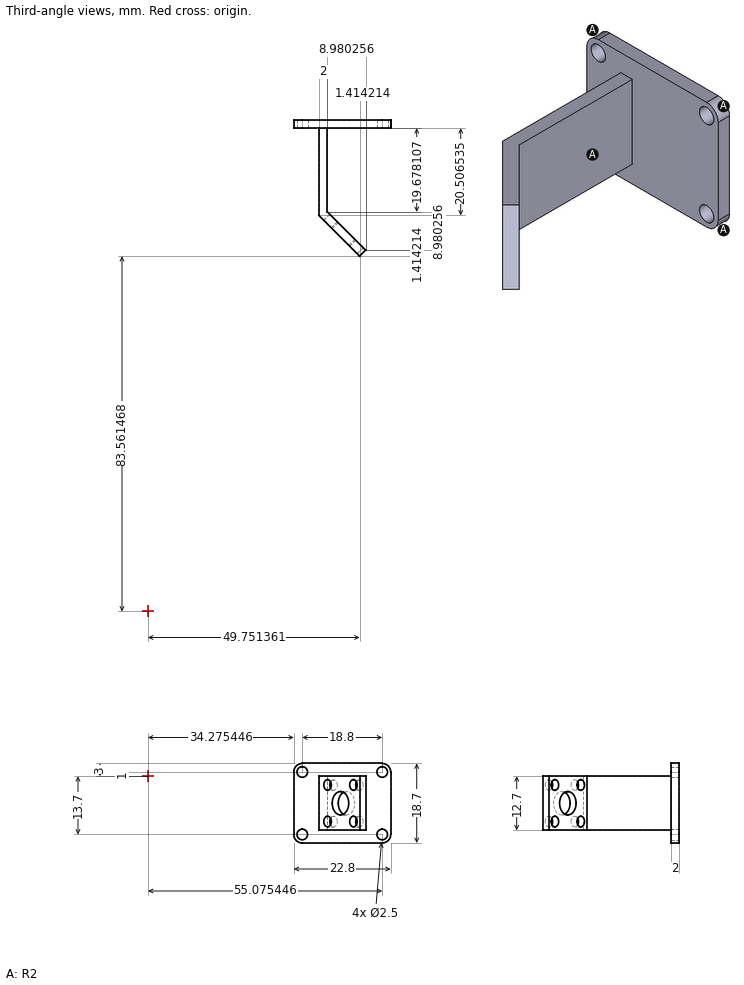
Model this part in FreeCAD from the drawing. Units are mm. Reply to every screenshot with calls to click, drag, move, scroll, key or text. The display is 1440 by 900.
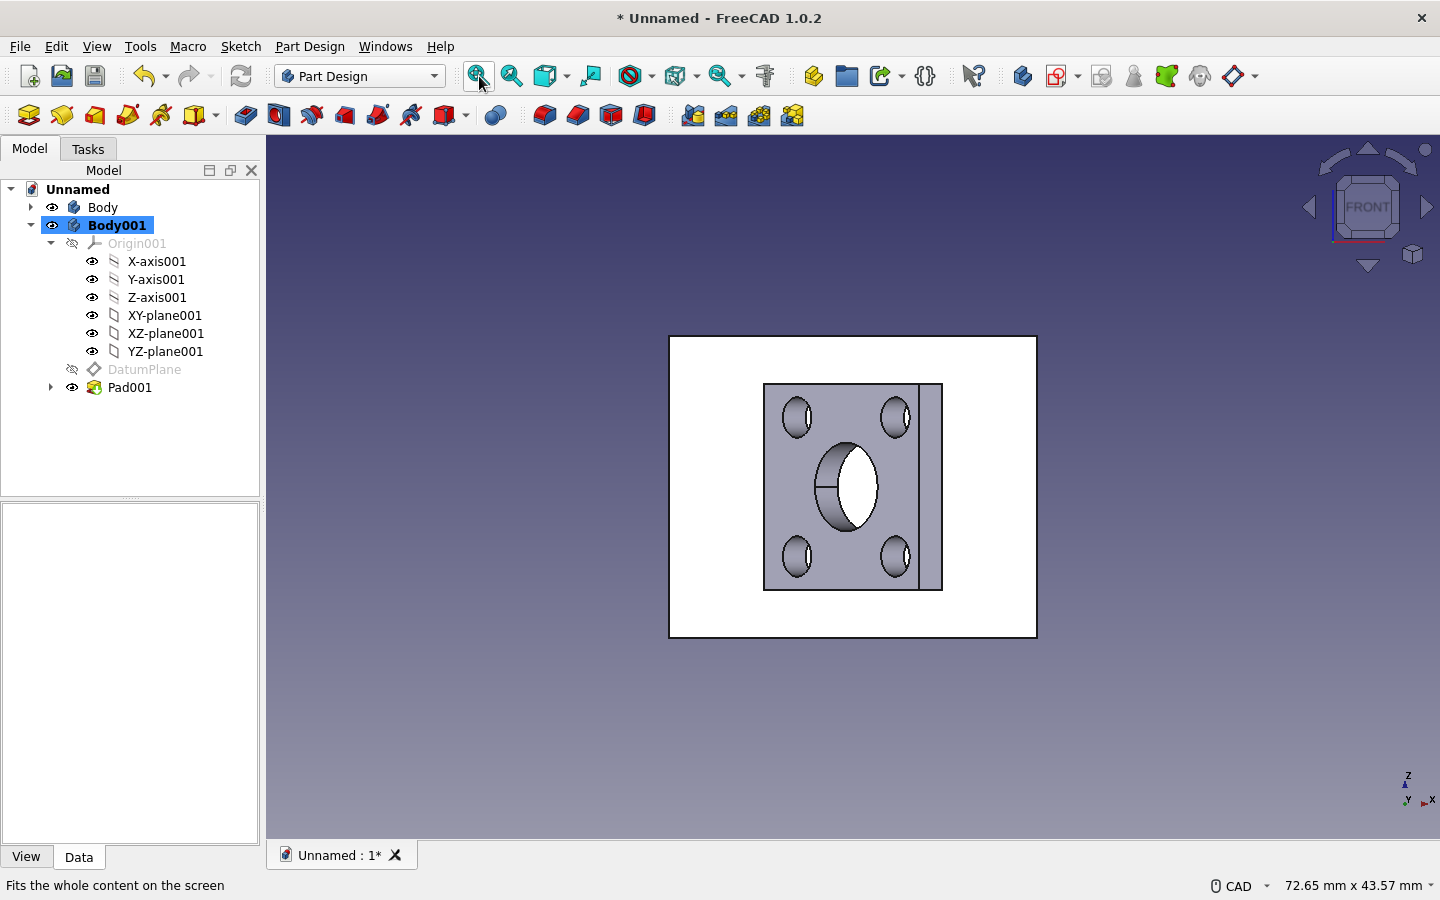
key(0)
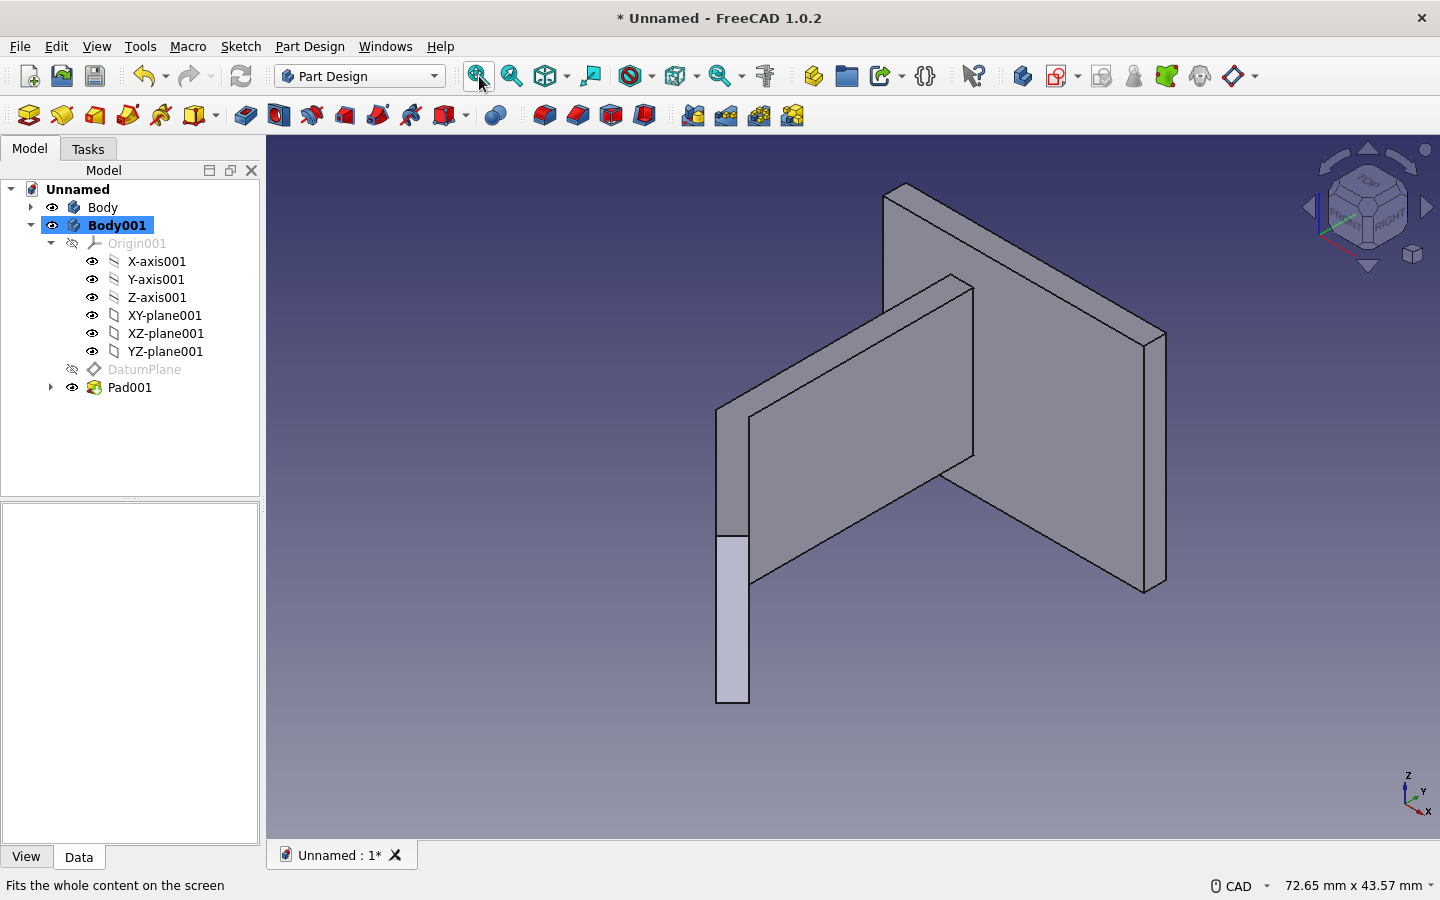
click(1155, 339)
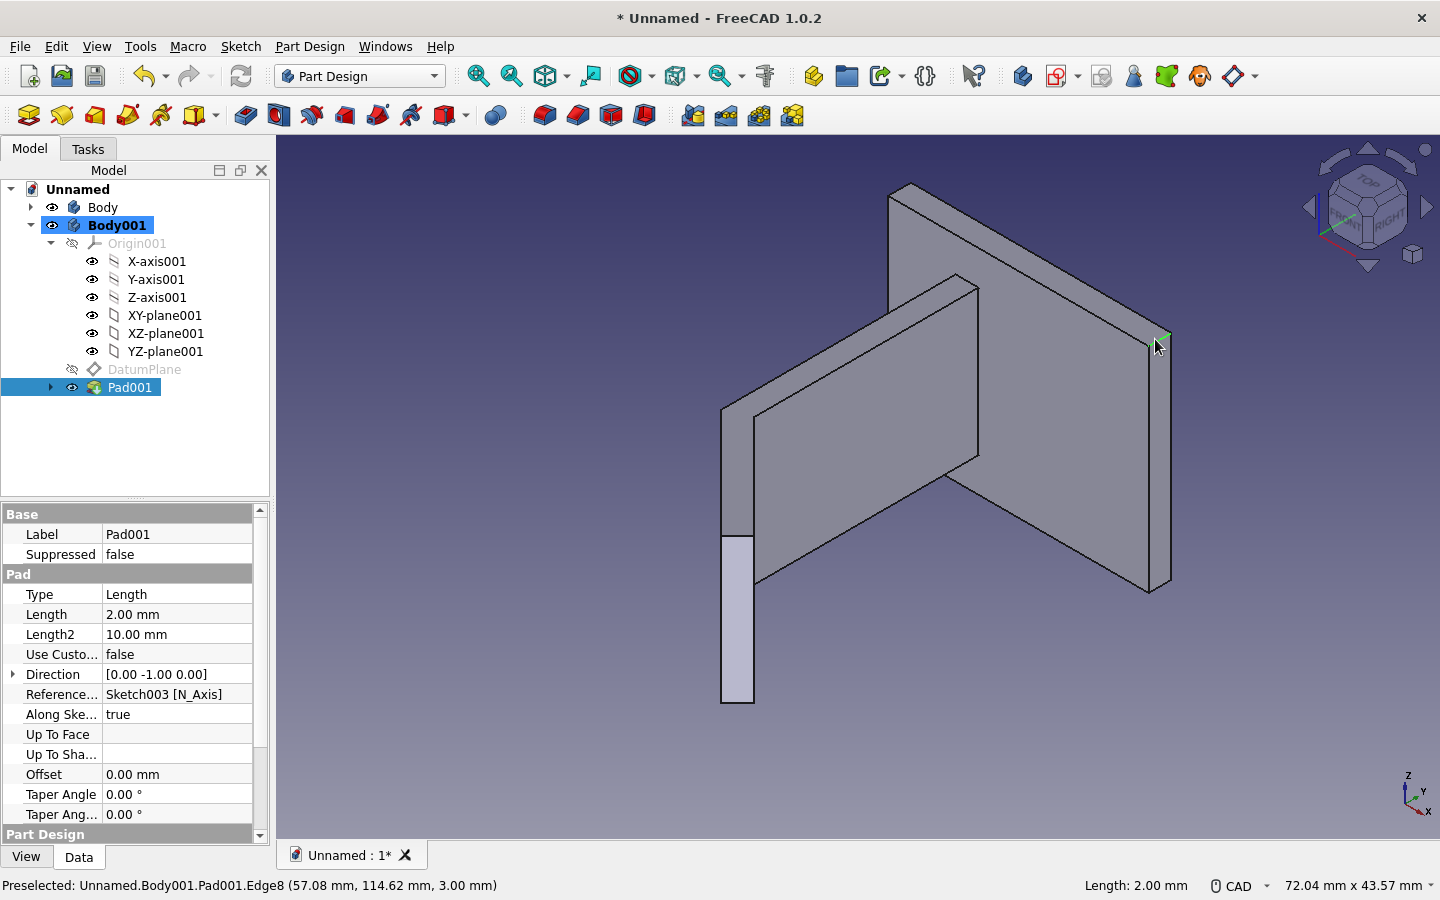
key(2)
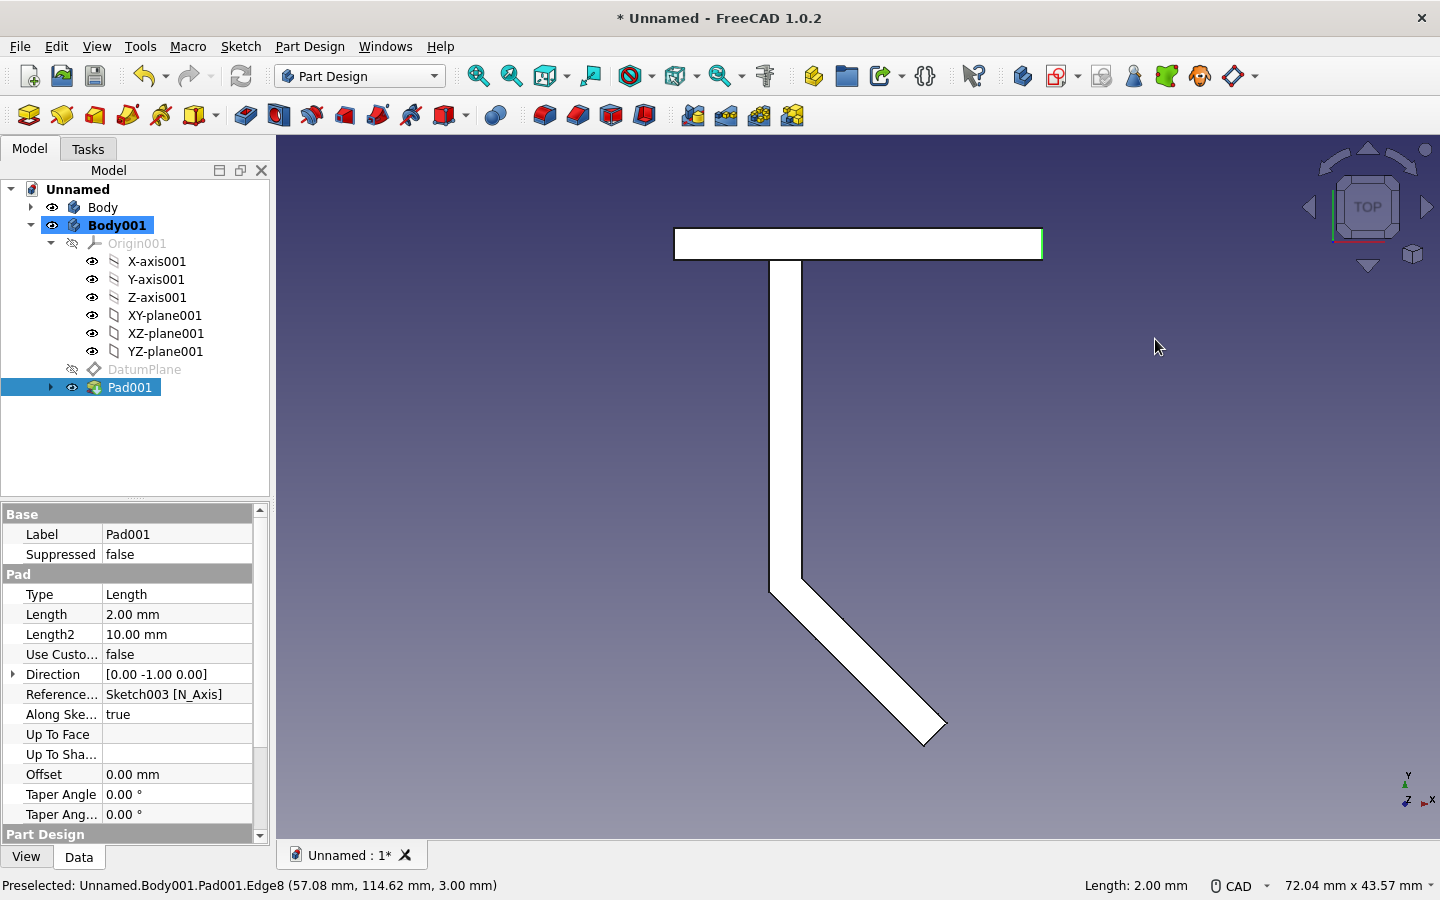
key(v)
key(f)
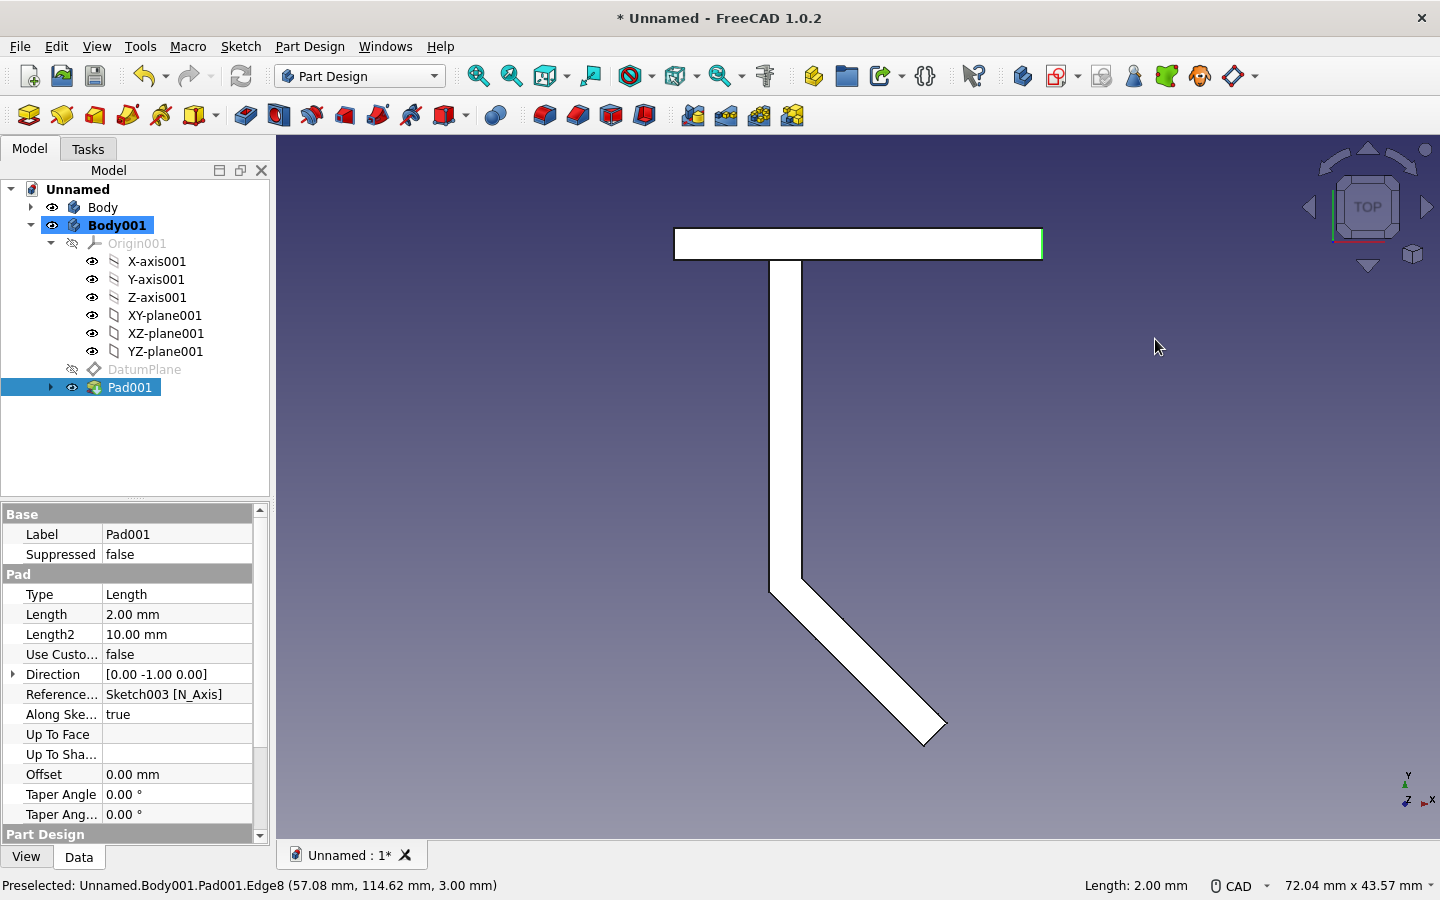
click(674, 243, ctrl)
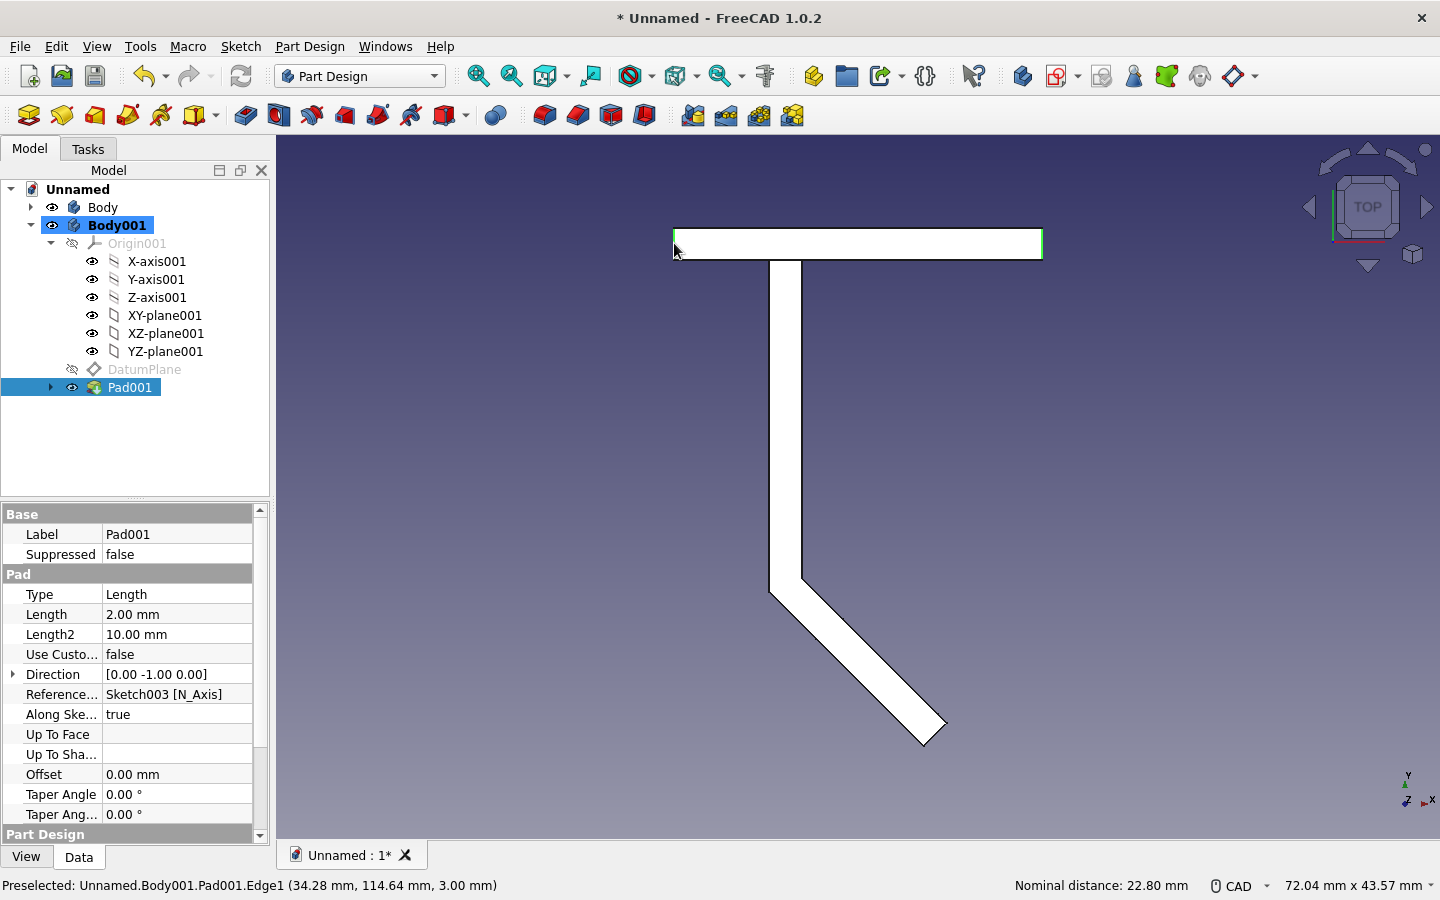
key(1)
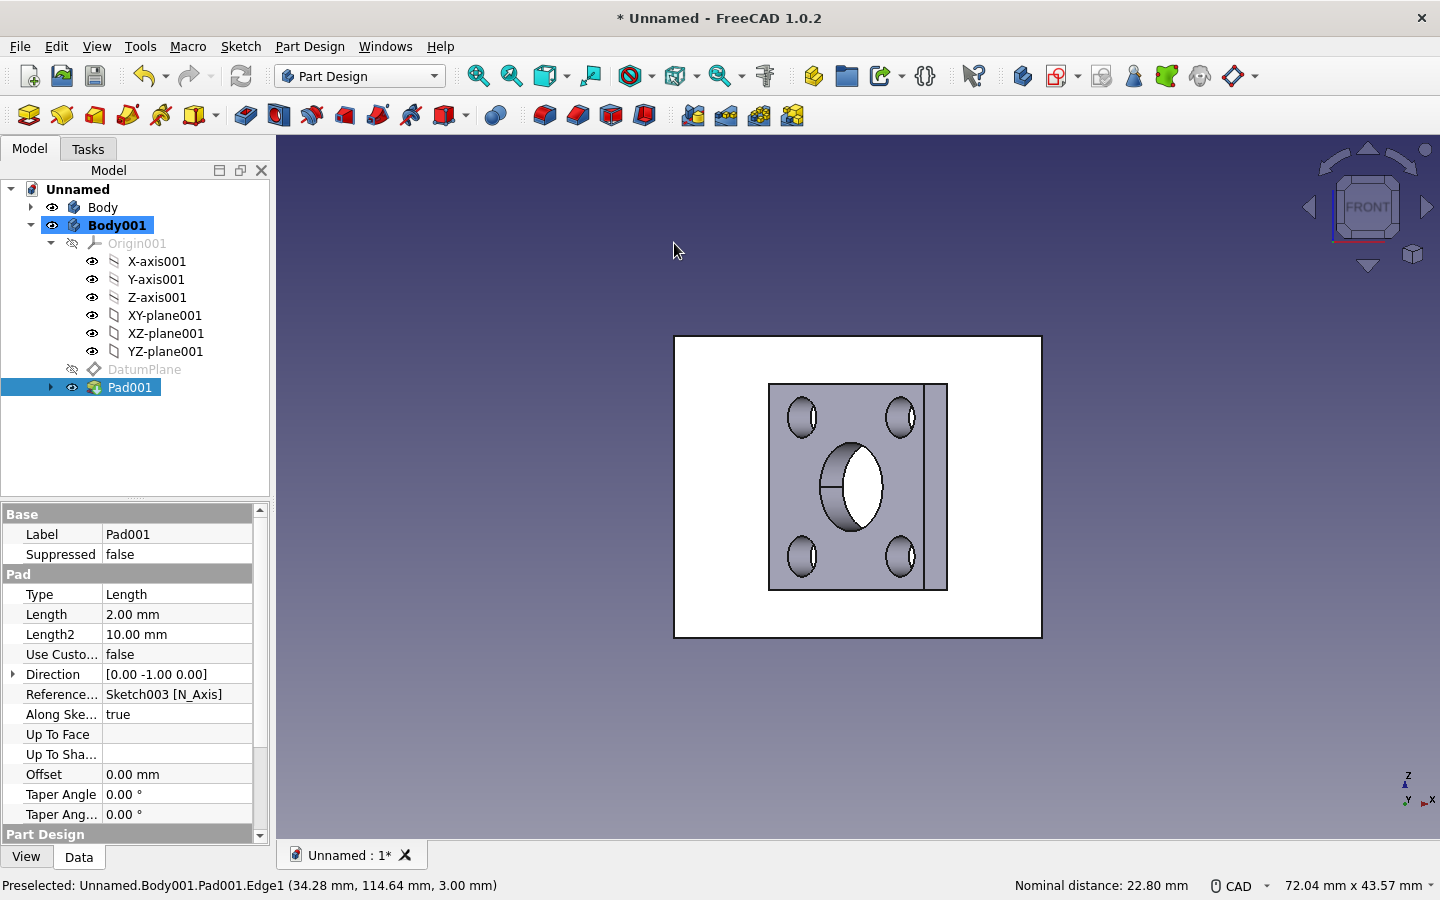
click(479, 76)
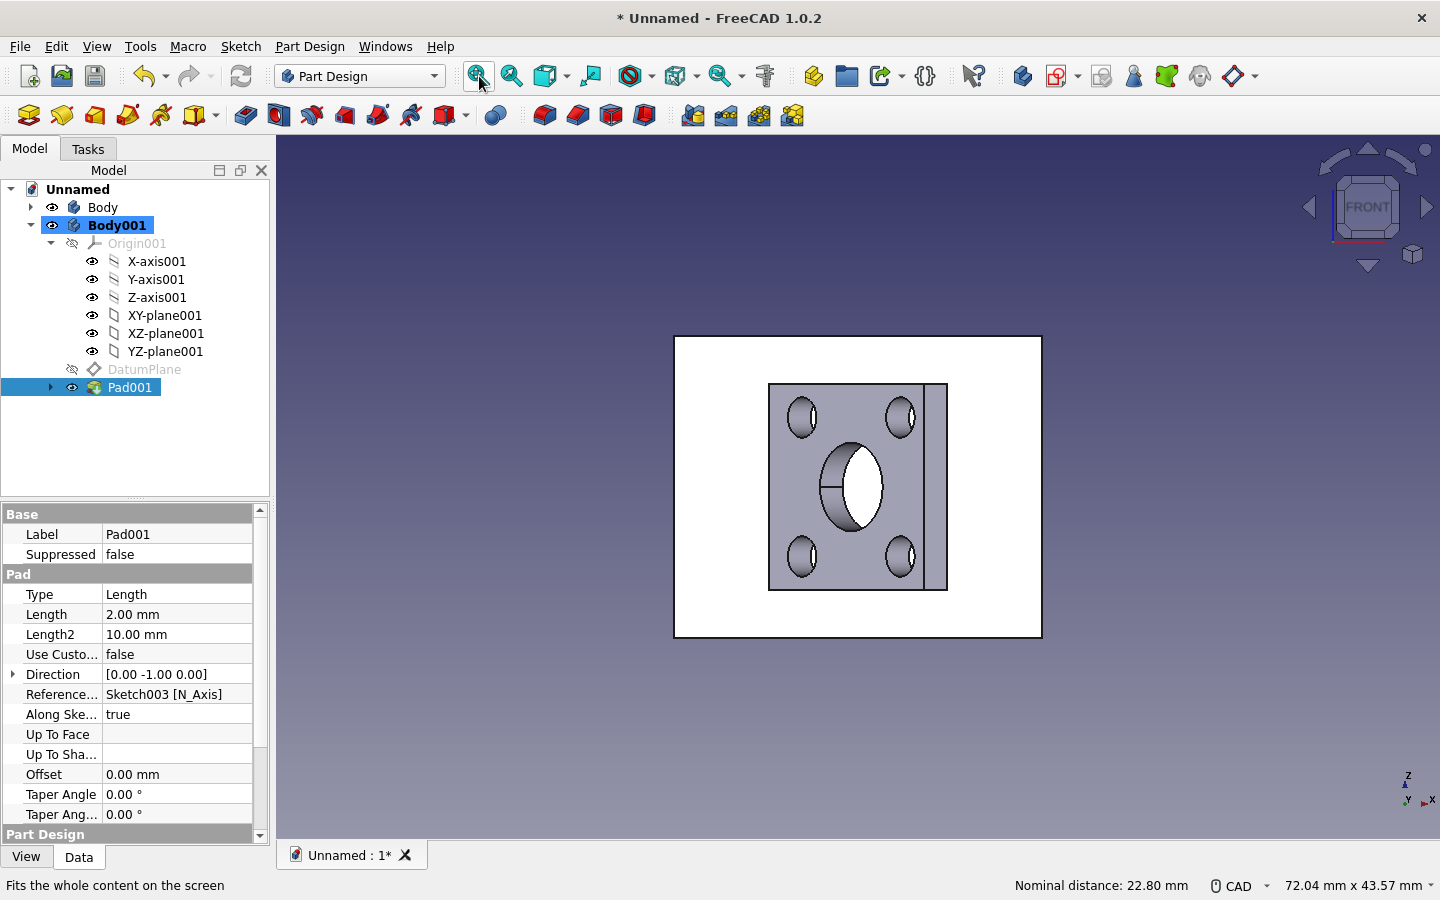
key(3)